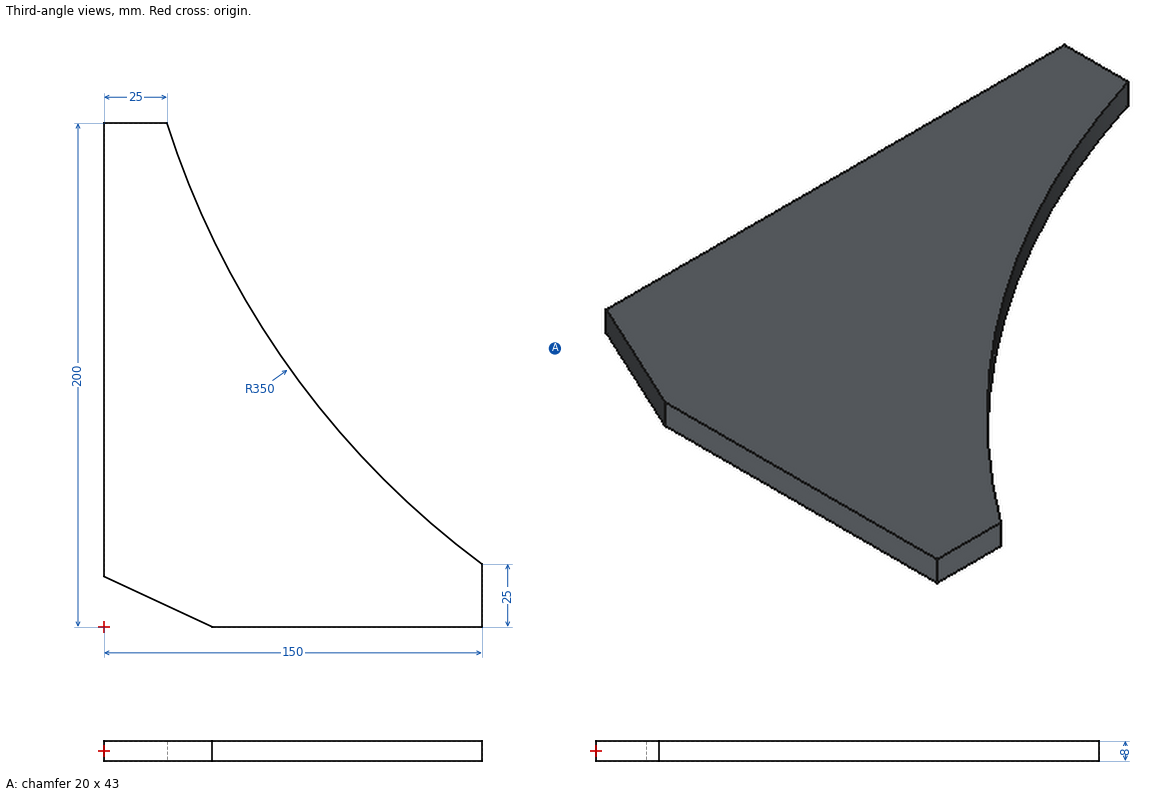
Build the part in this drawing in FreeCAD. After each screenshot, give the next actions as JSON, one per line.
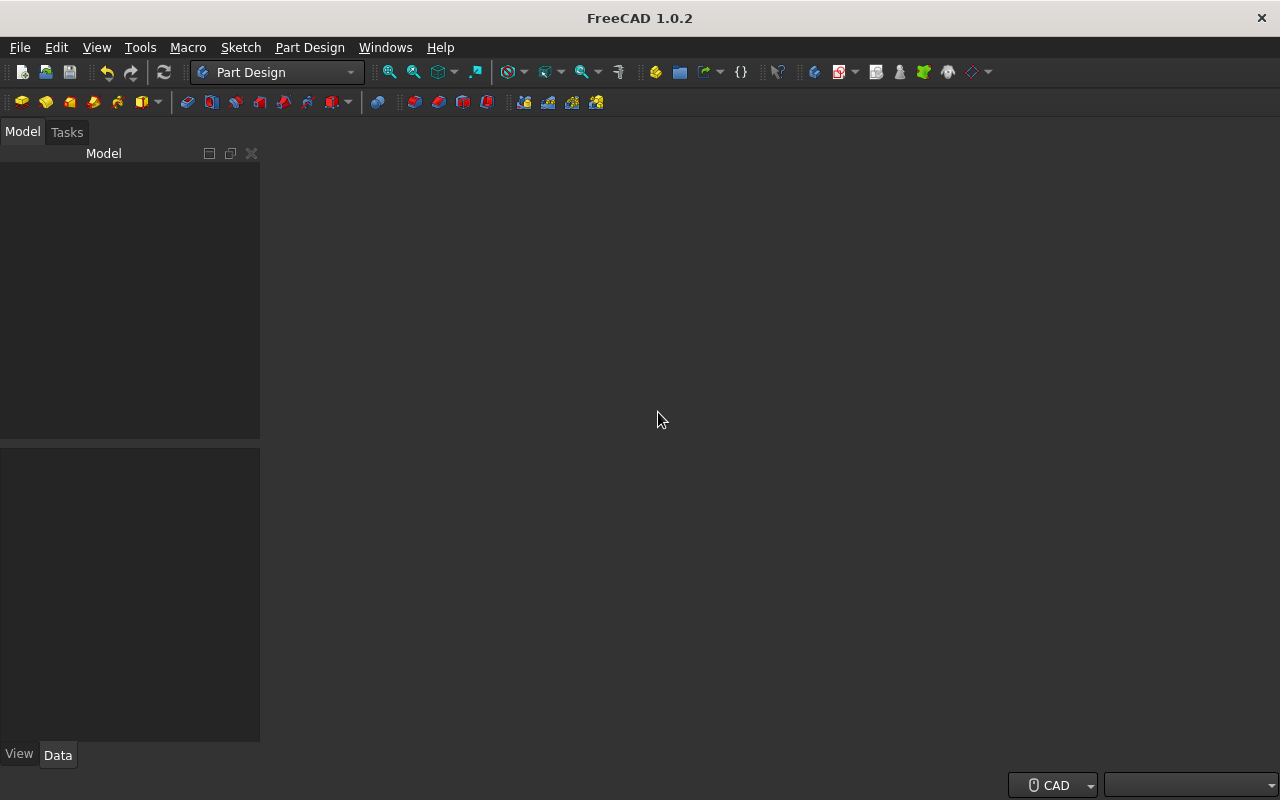
{"action": "left_click", "coordinate": [22, 72]}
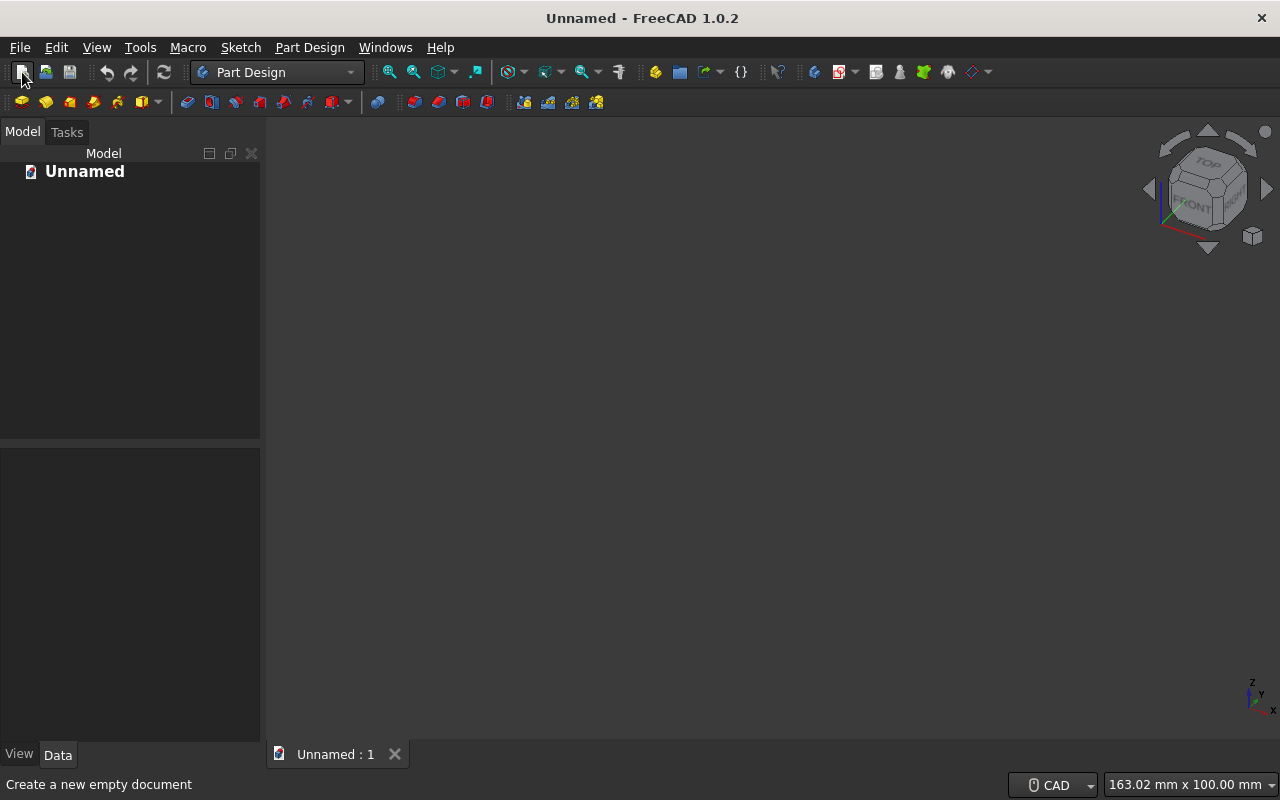
{"action": "left_click", "coordinate": [840, 72]}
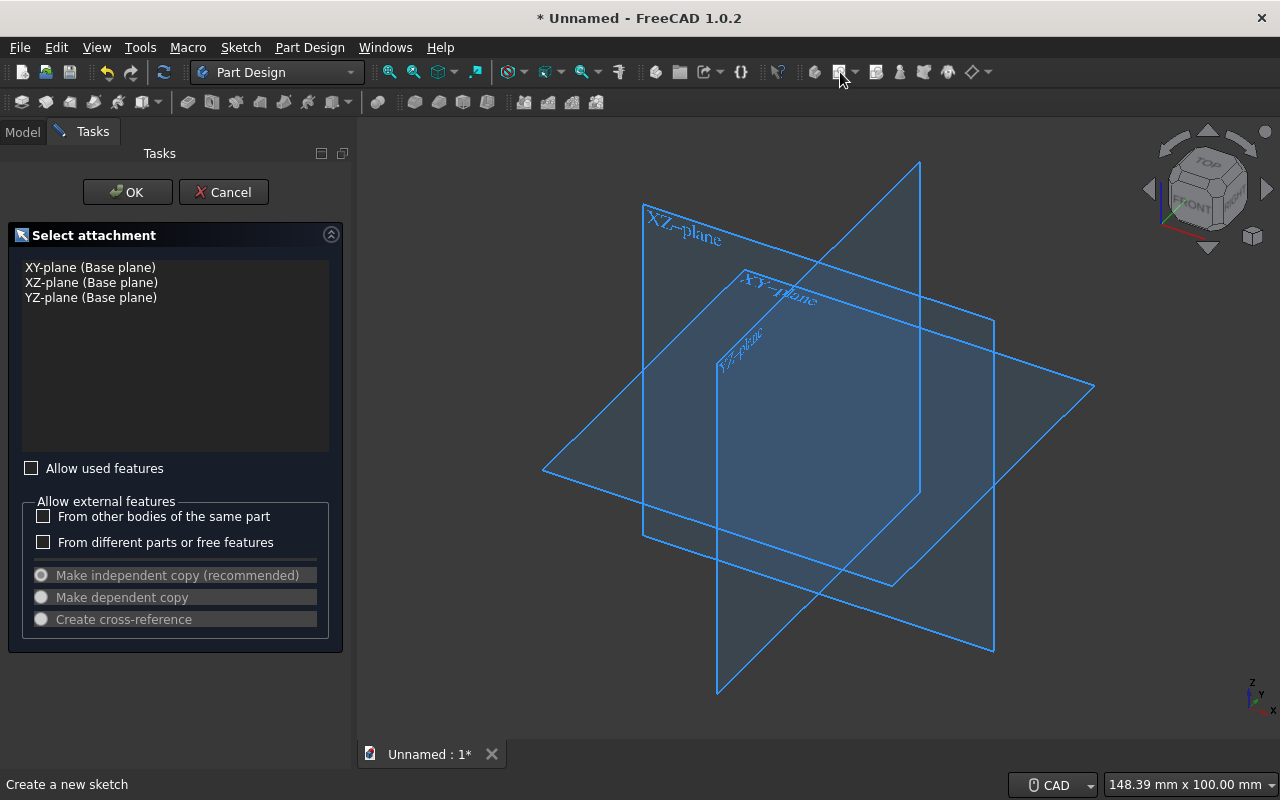
{"action": "left_click", "coordinate": [82, 268]}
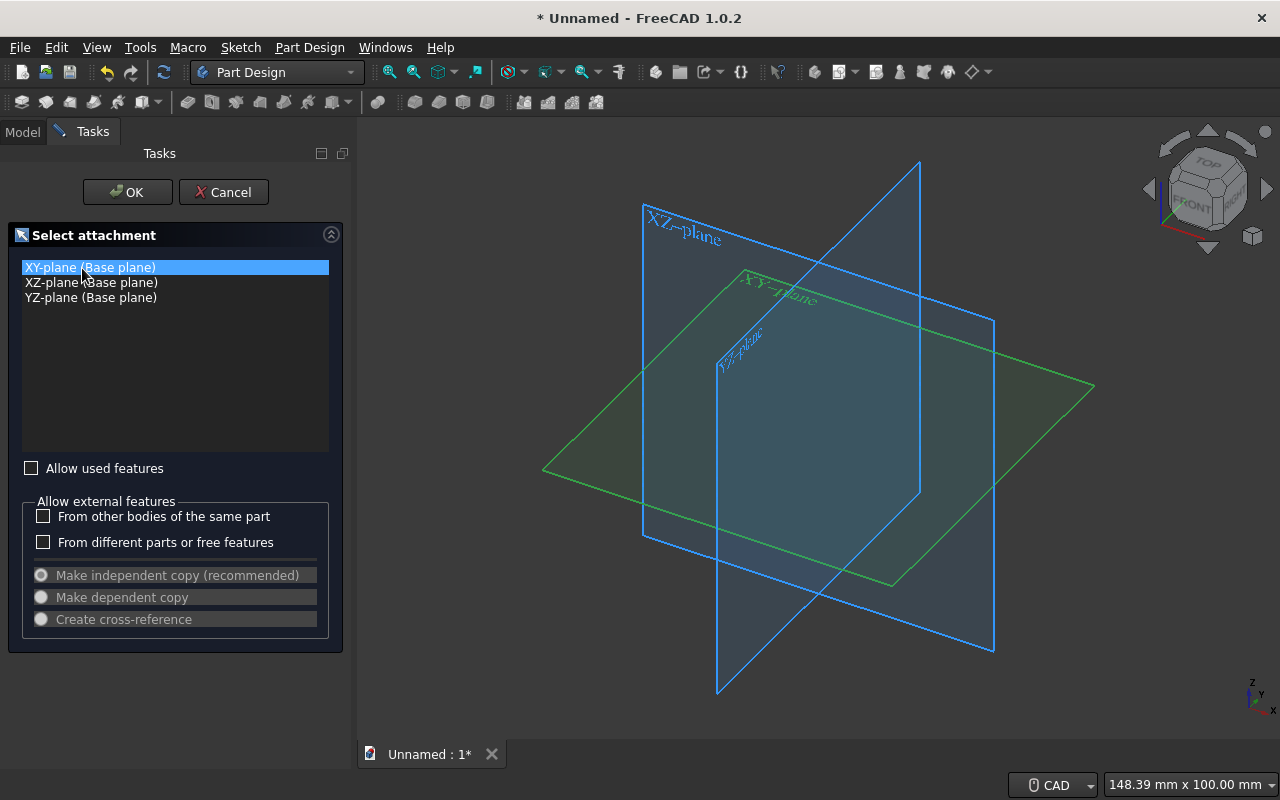
{"action": "left_click", "coordinate": [128, 192]}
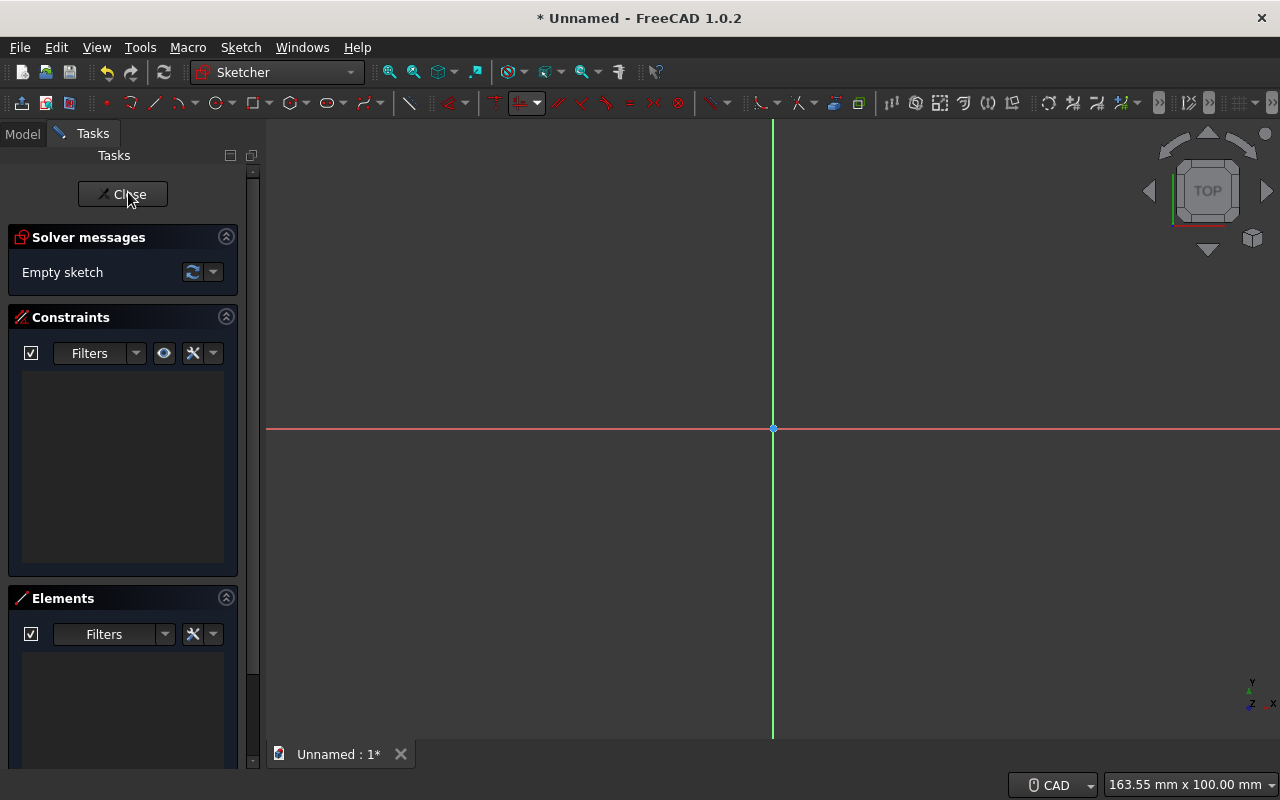
{"action": "scroll", "coordinate": [475, 696], "scroll_direction": "down", "scroll_amount": 6}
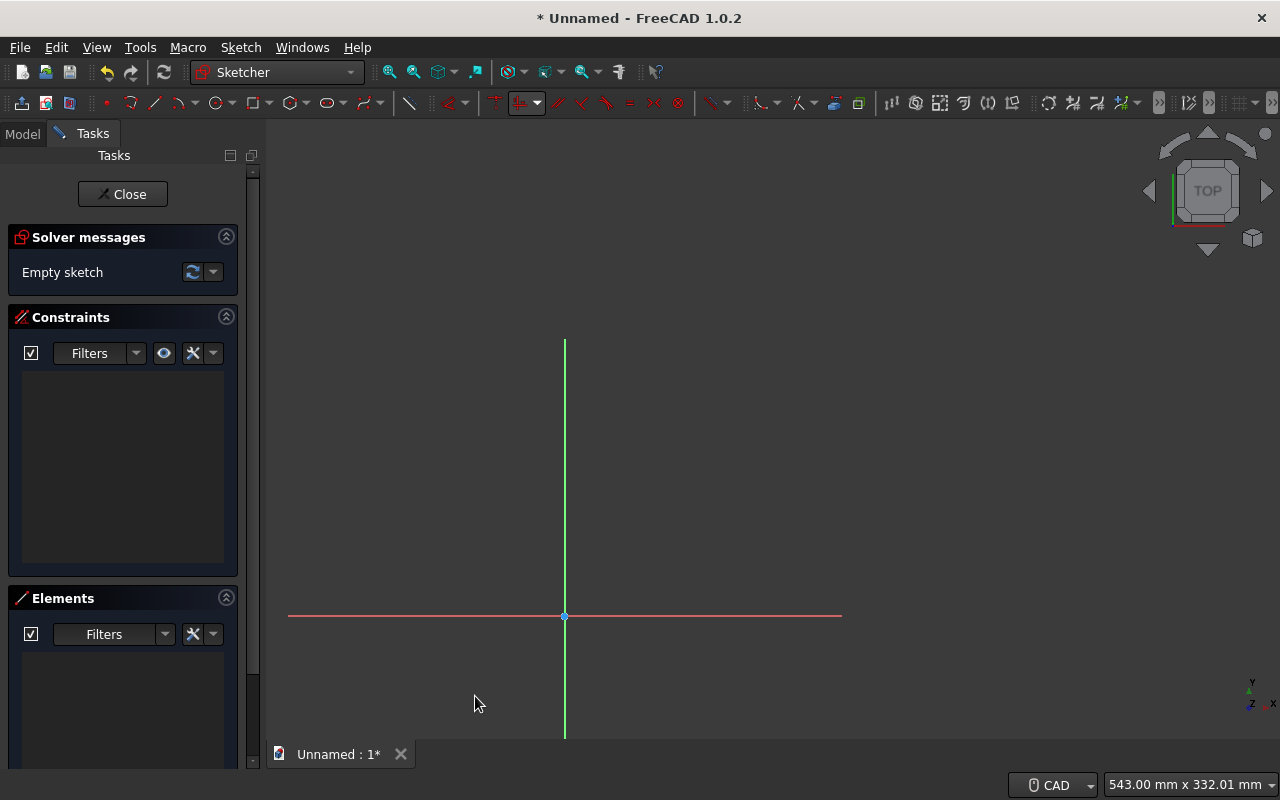
{"action": "left_click", "coordinate": [132, 104]}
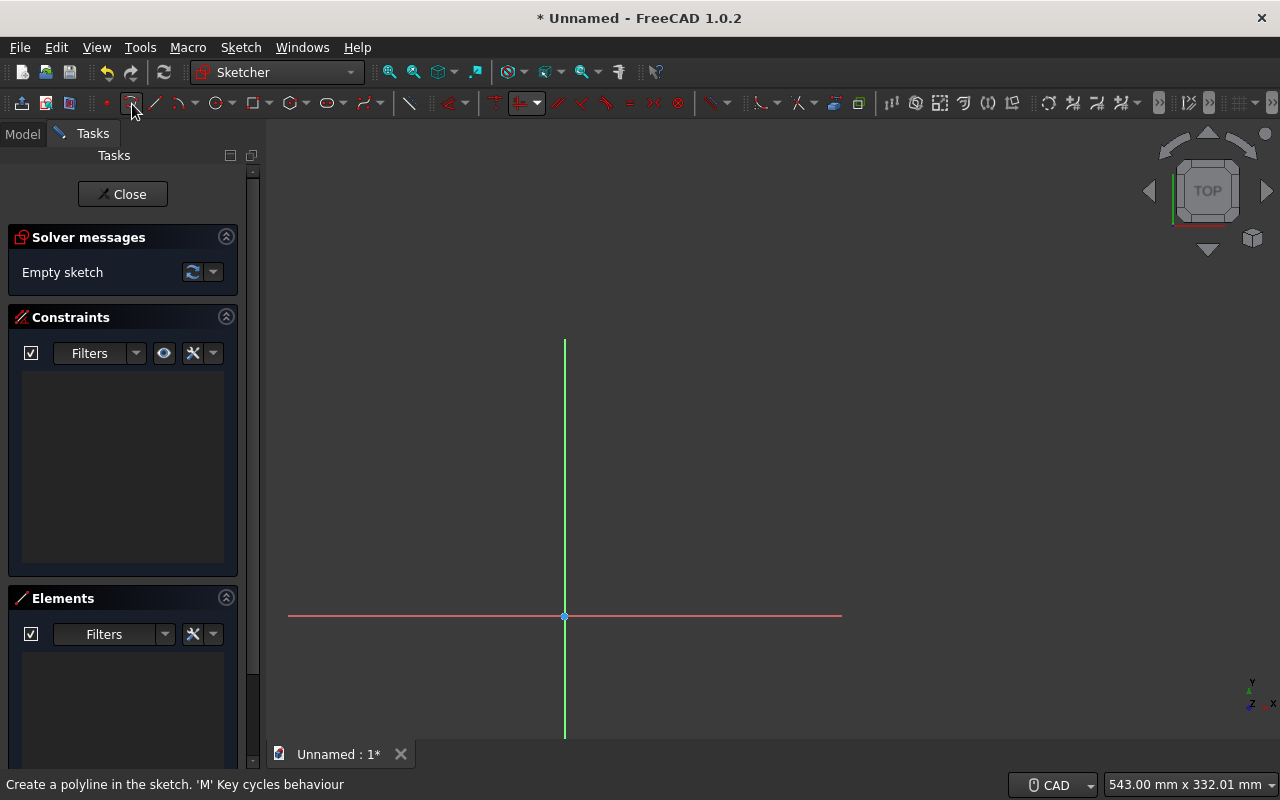
{"action": "left_click", "coordinate": [565, 616]}
{"action": "left_click", "coordinate": [845, 607]}
{"action": "left_click", "coordinate": [845, 570]}
{"action": "left_click", "coordinate": [612, 243]}
{"action": "left_click", "coordinate": [574, 243]}
{"action": "left_click", "coordinate": [565, 616]}
{"action": "key", "text": "Escape"}
{"action": "key", "text": "Escape"}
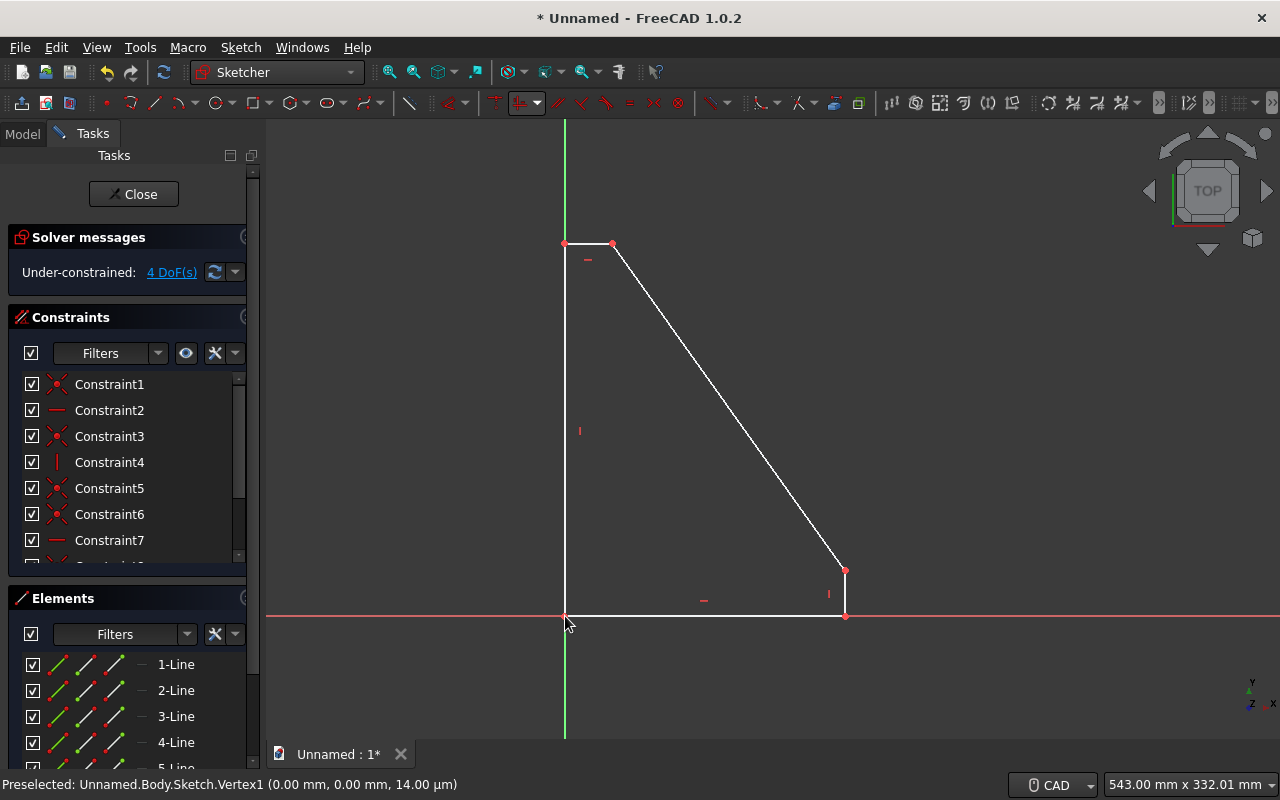
{"action": "key", "text": "d"}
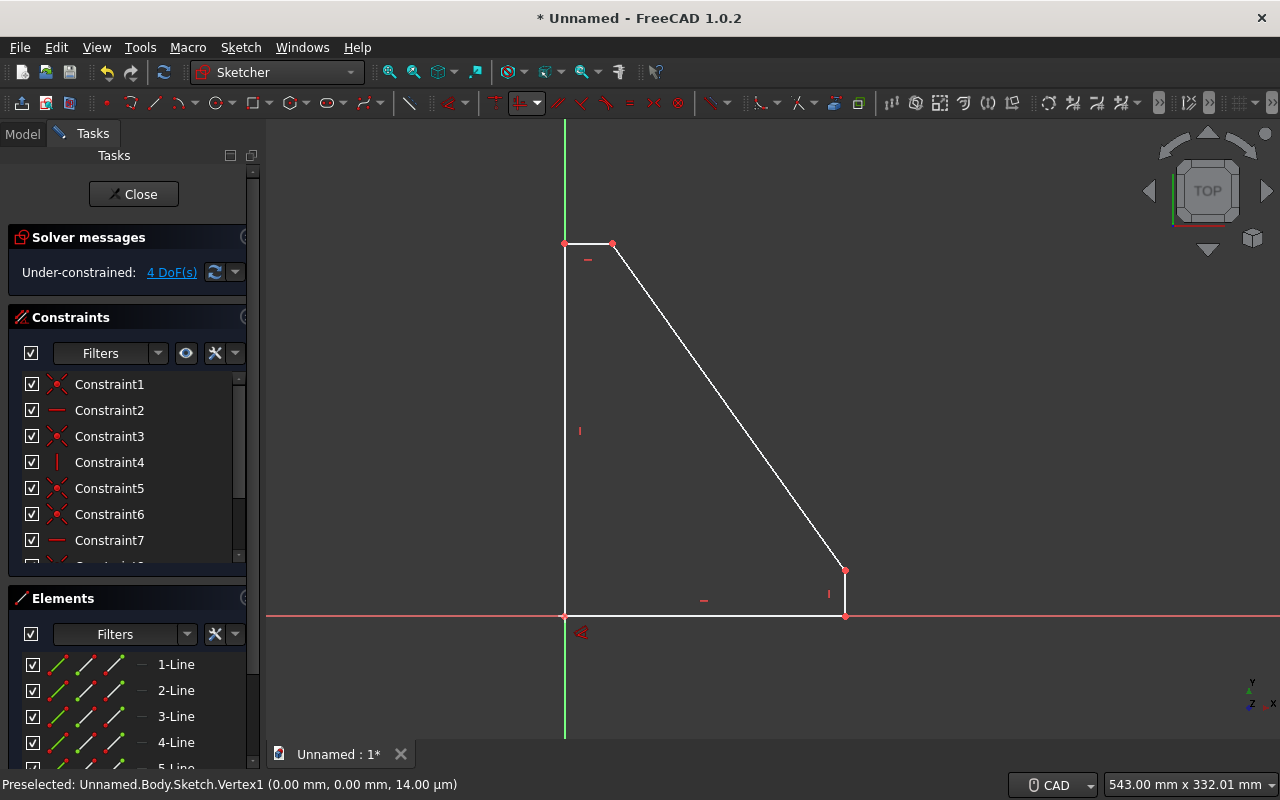
{"action": "left_click", "coordinate": [845, 603]}
{"action": "left_click", "coordinate": [879, 594]}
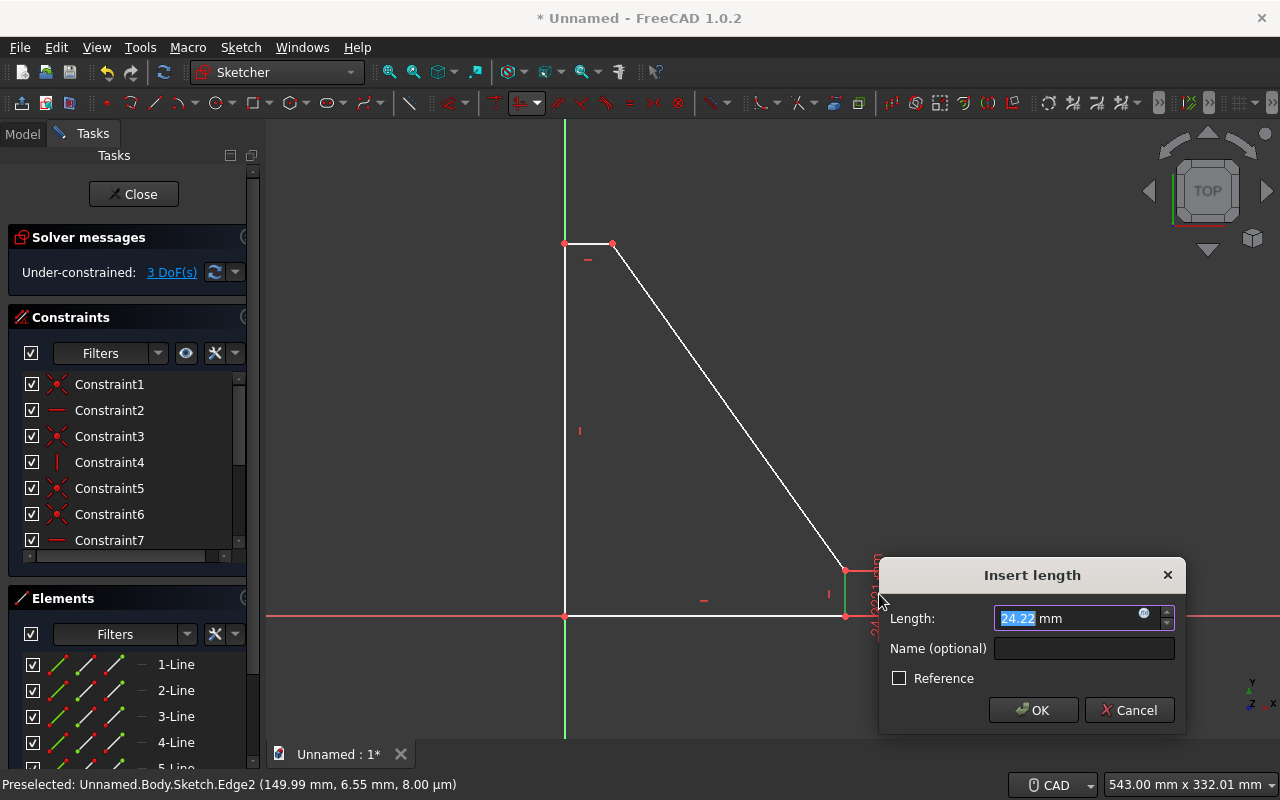
{"action": "type", "text": "25"}
{"action": "key", "text": "Return"}